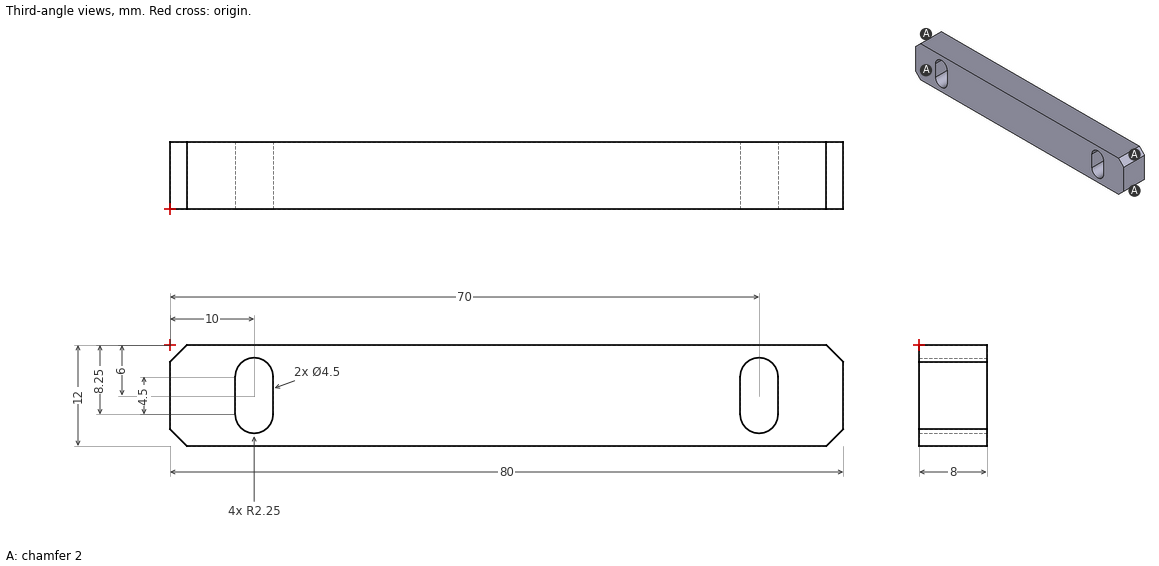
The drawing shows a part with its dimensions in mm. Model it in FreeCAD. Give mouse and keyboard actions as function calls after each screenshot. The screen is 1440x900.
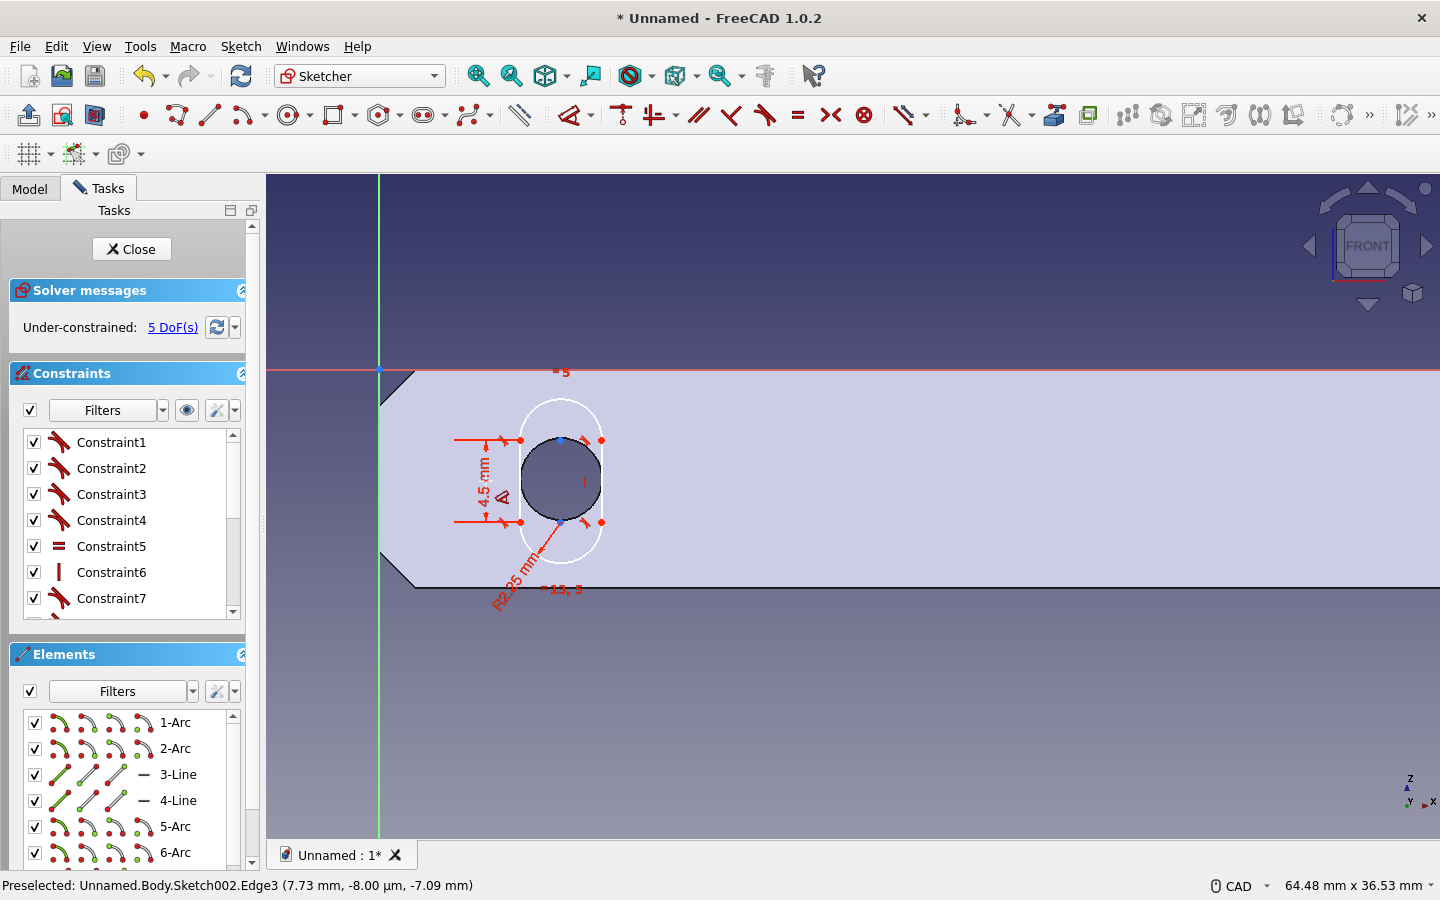
scroll(477, 556, down, 3)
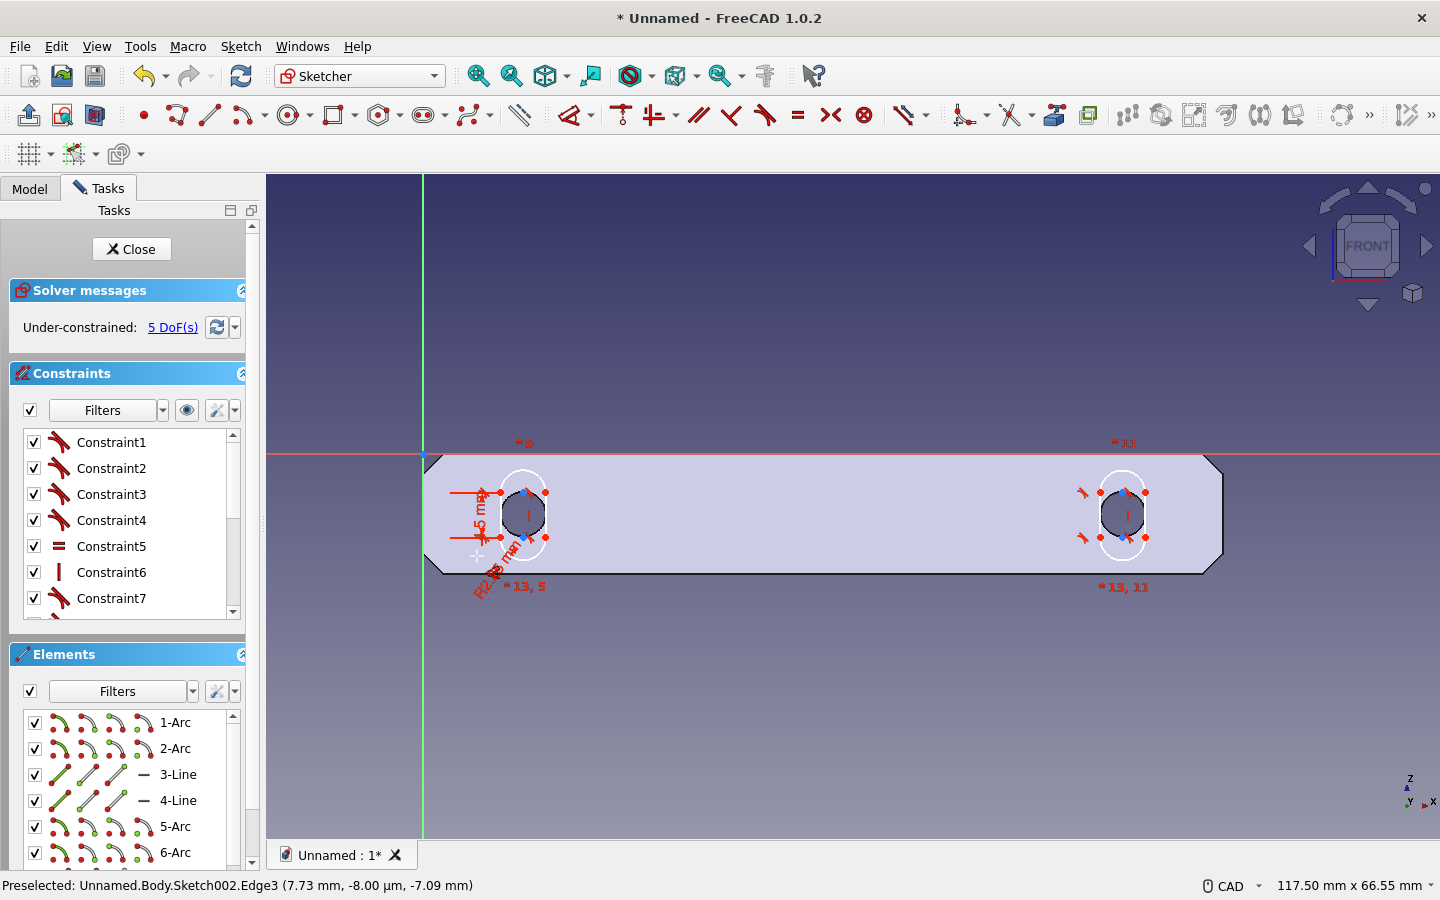
click(1100, 525)
click(1066, 516)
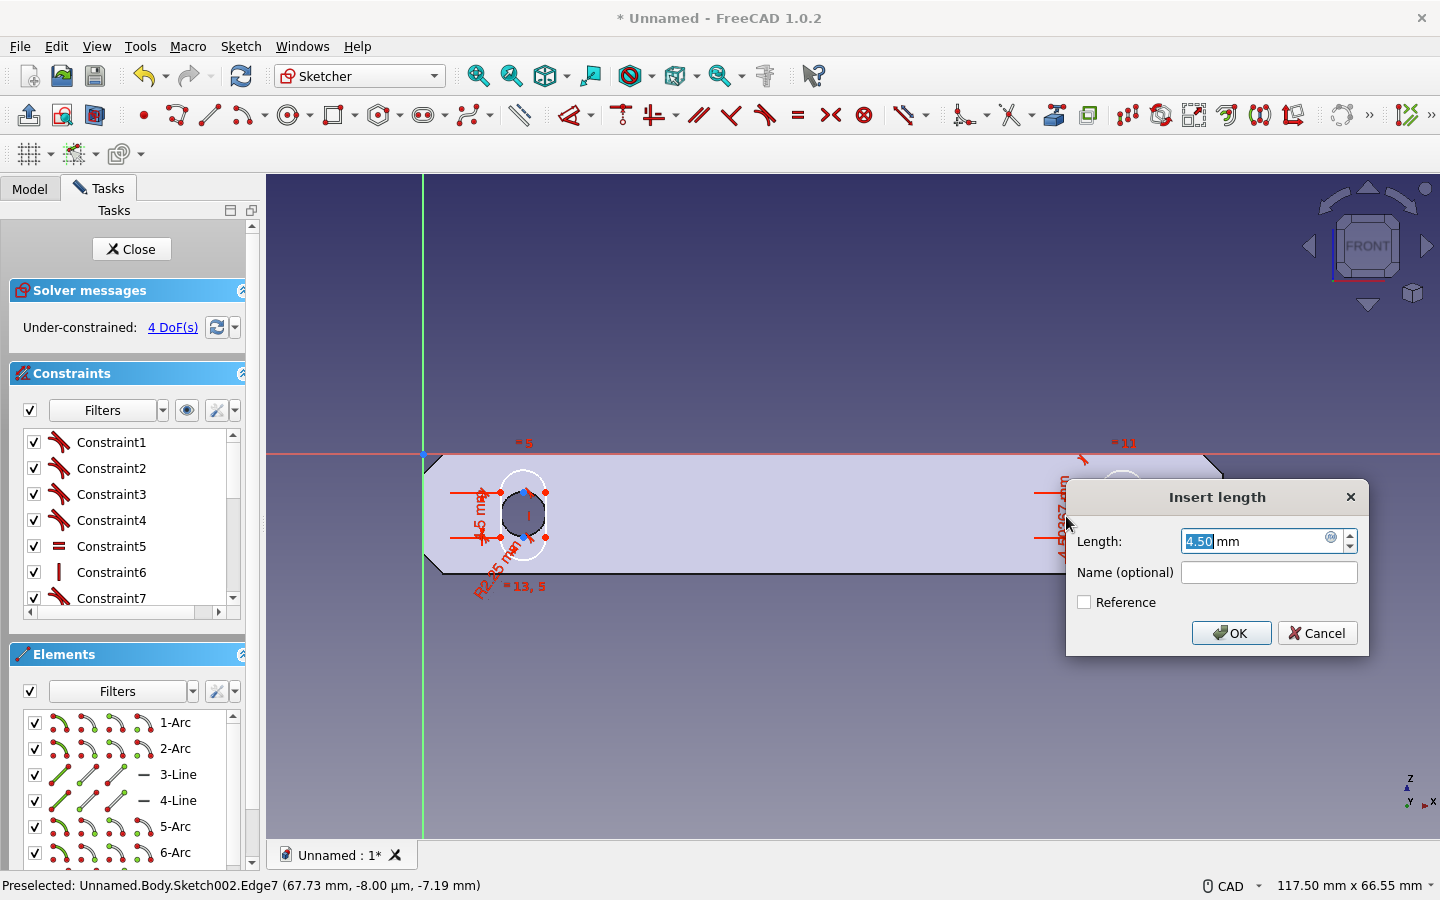
text(4.5)
key(Return)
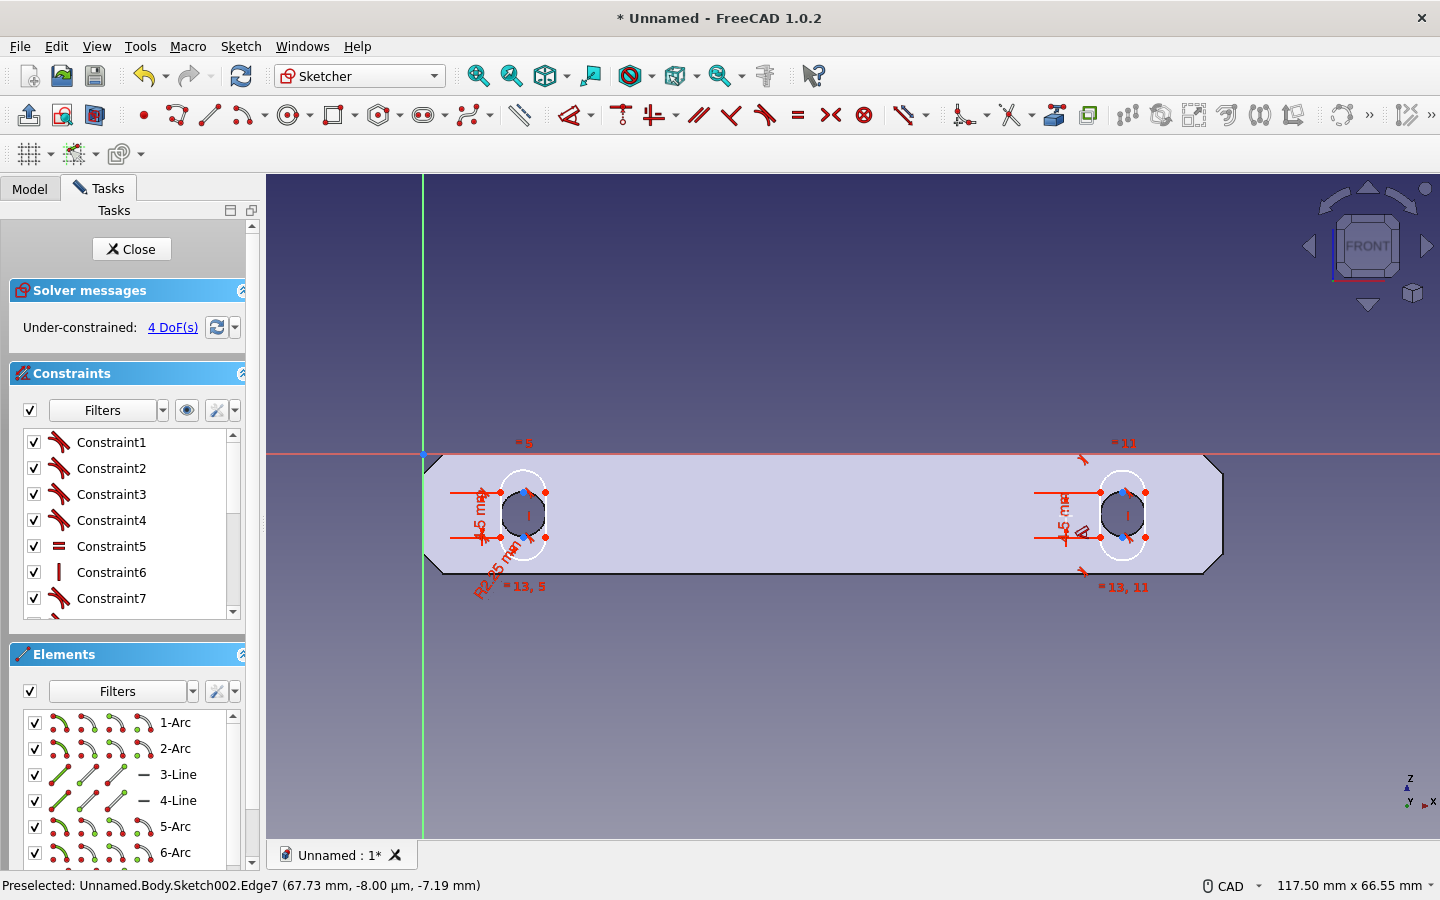
click(523, 538)
click(473, 420)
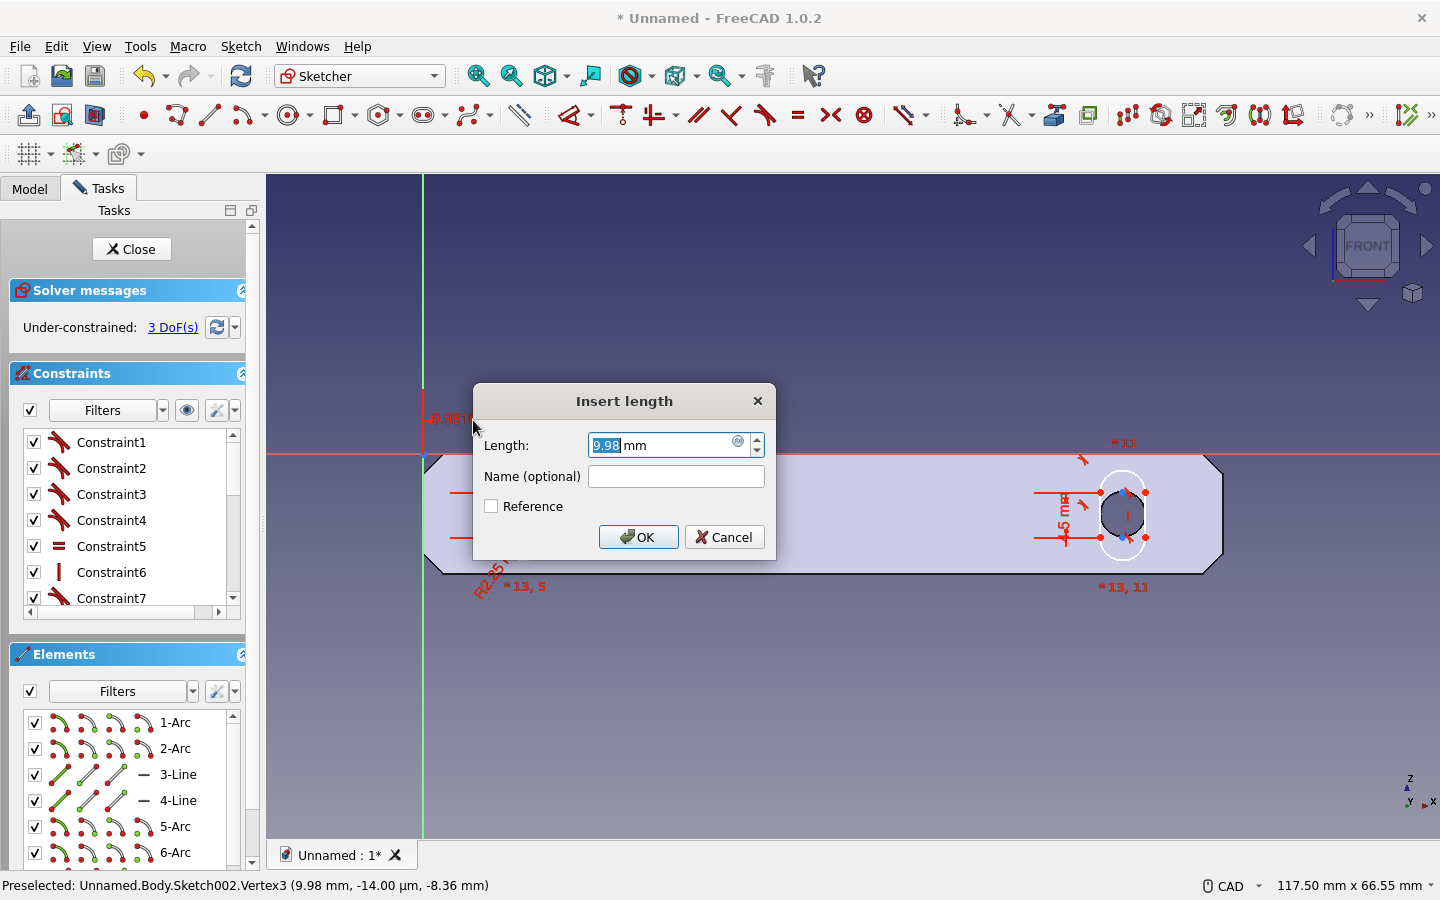
text(10)
key(Return)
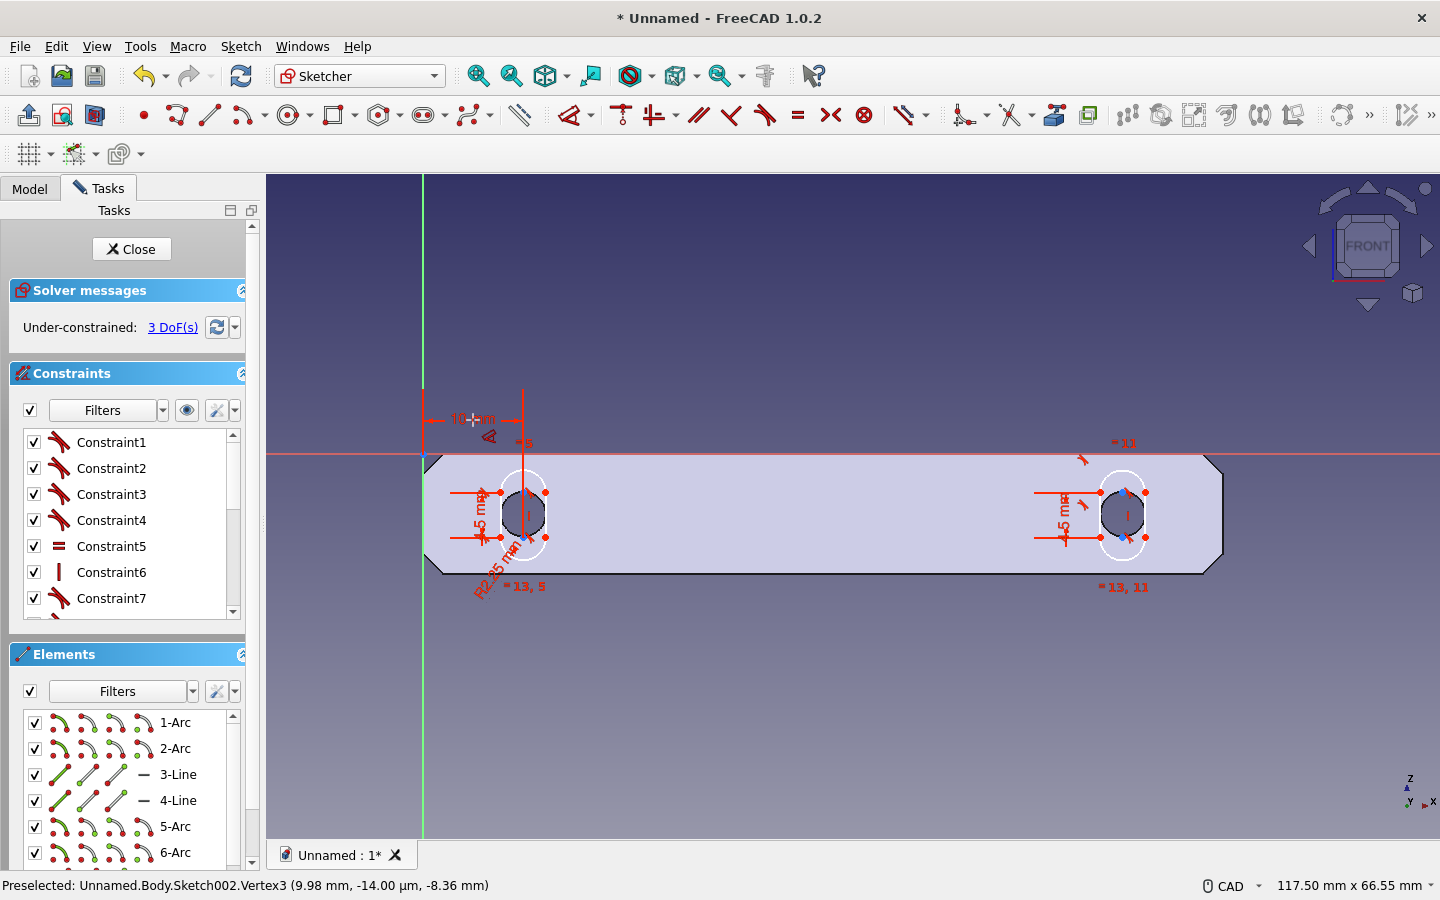
click(1123, 538)
click(773, 420)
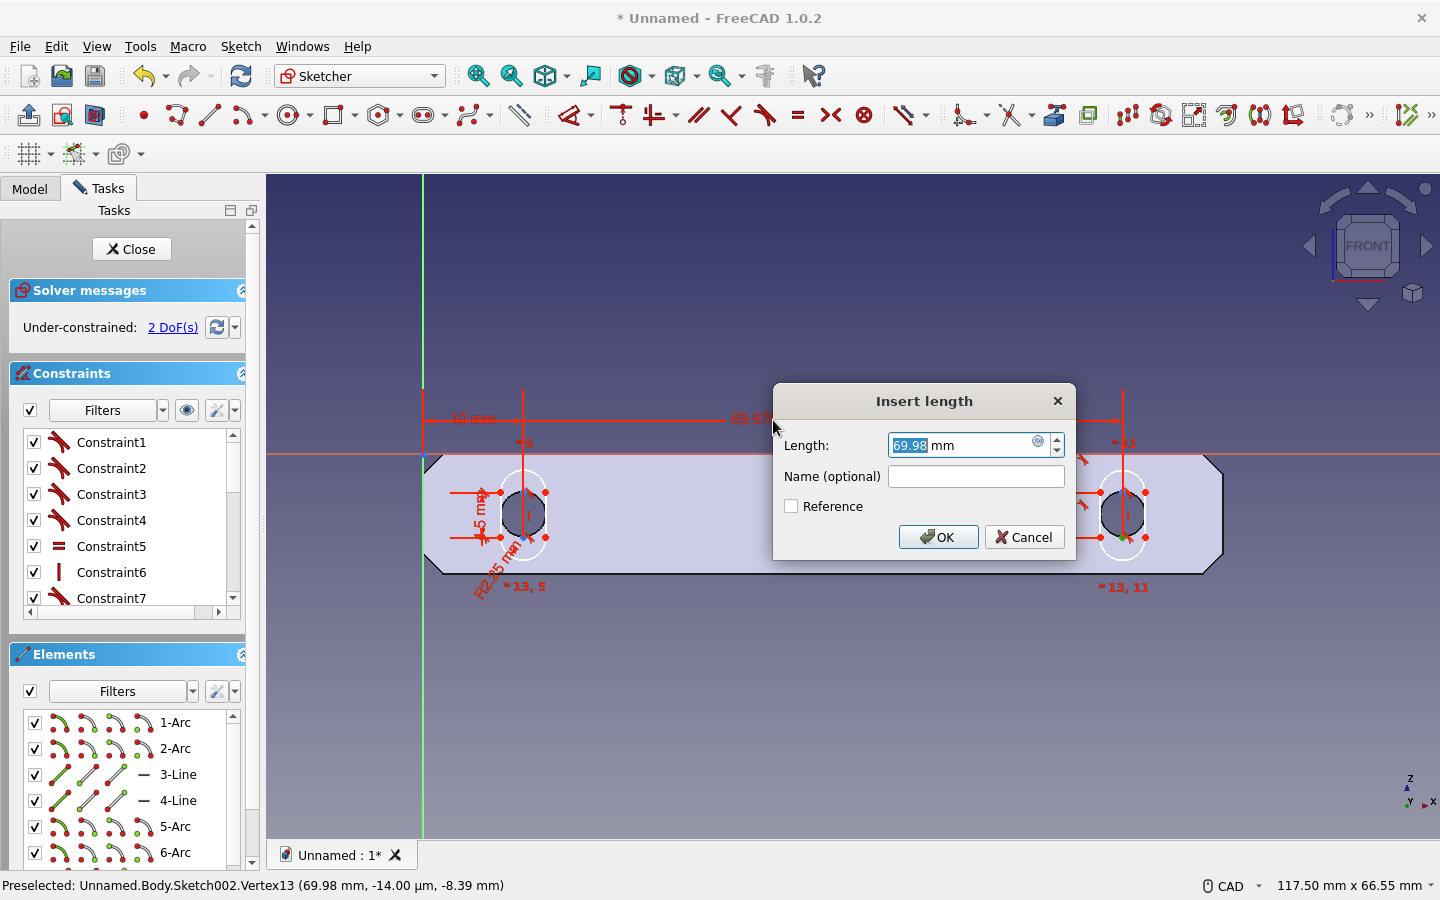
text(70)
key(Return)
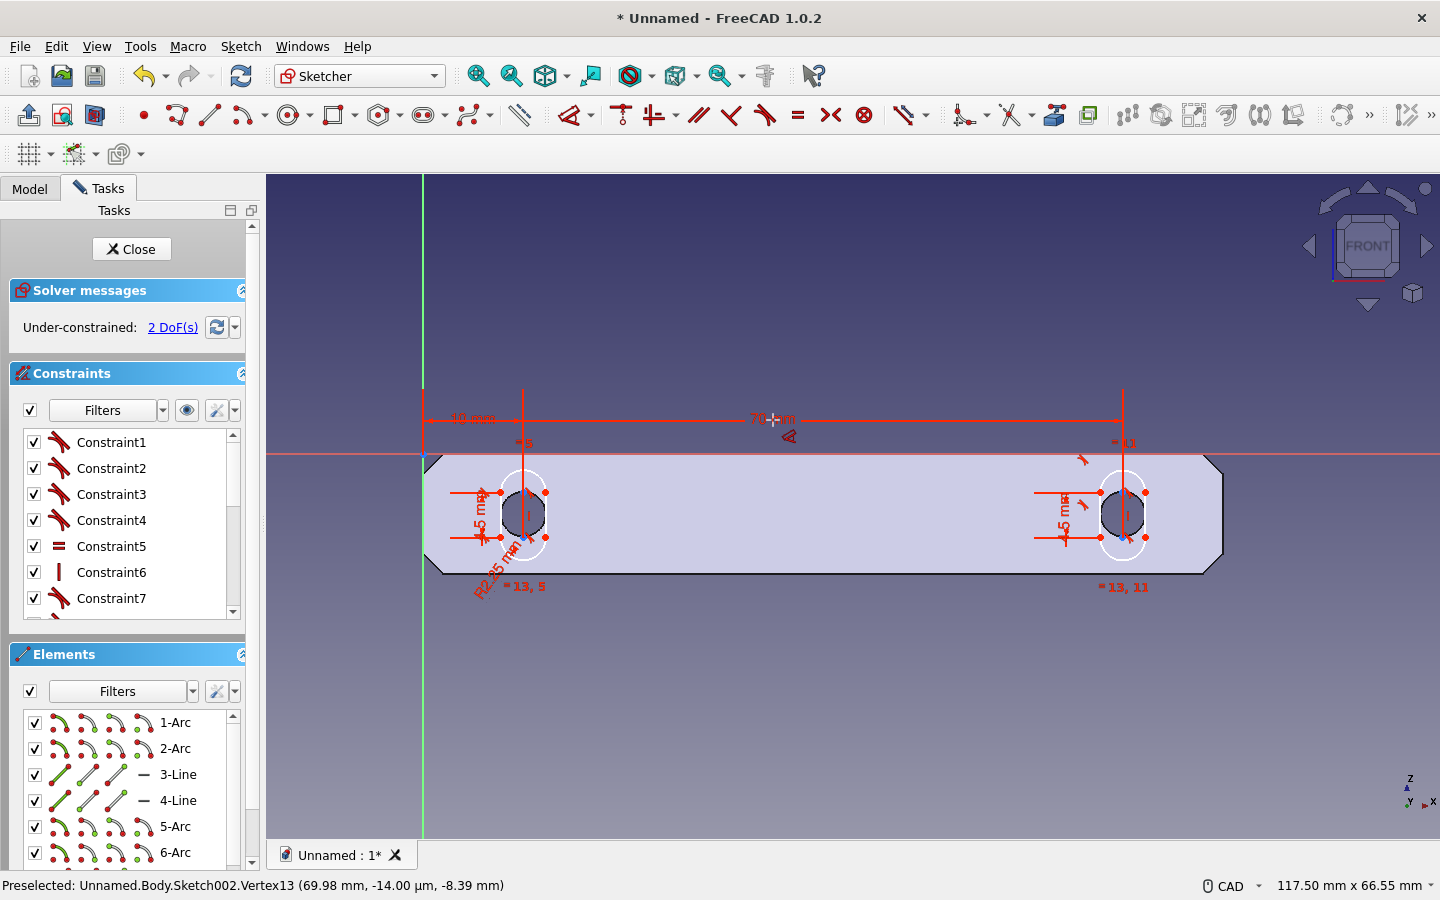
click(501, 538)
click(389, 496)